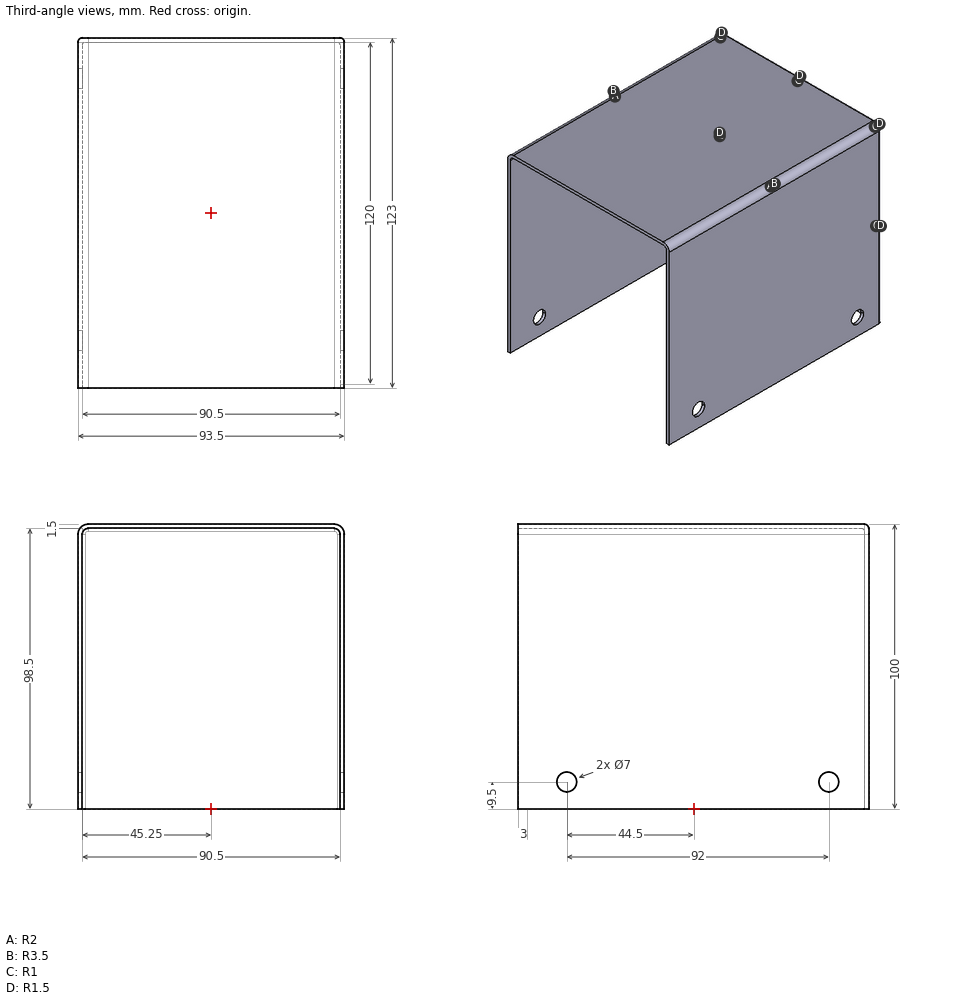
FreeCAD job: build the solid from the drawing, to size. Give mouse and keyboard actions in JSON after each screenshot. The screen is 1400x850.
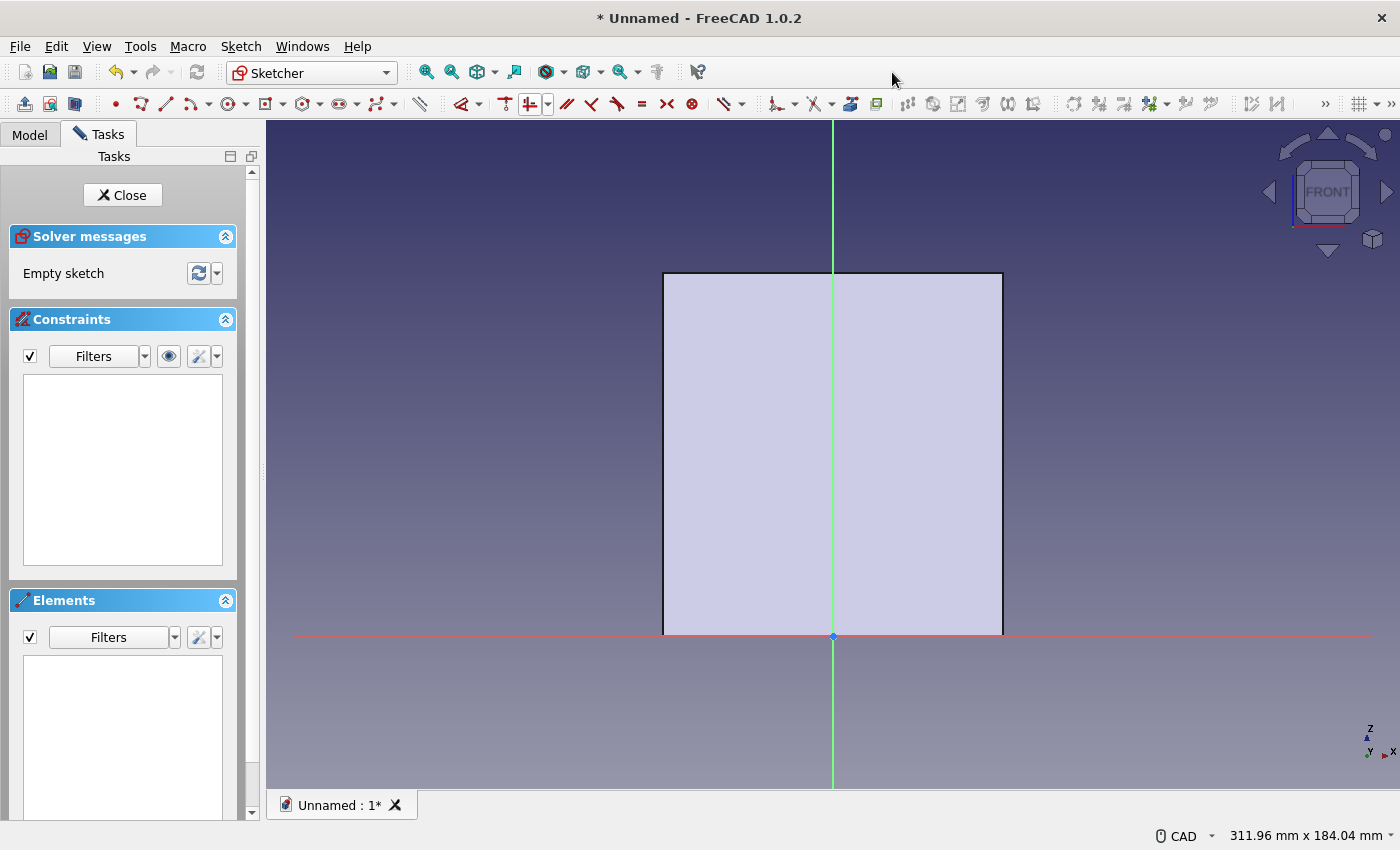
{"action": "key", "text": "g r"}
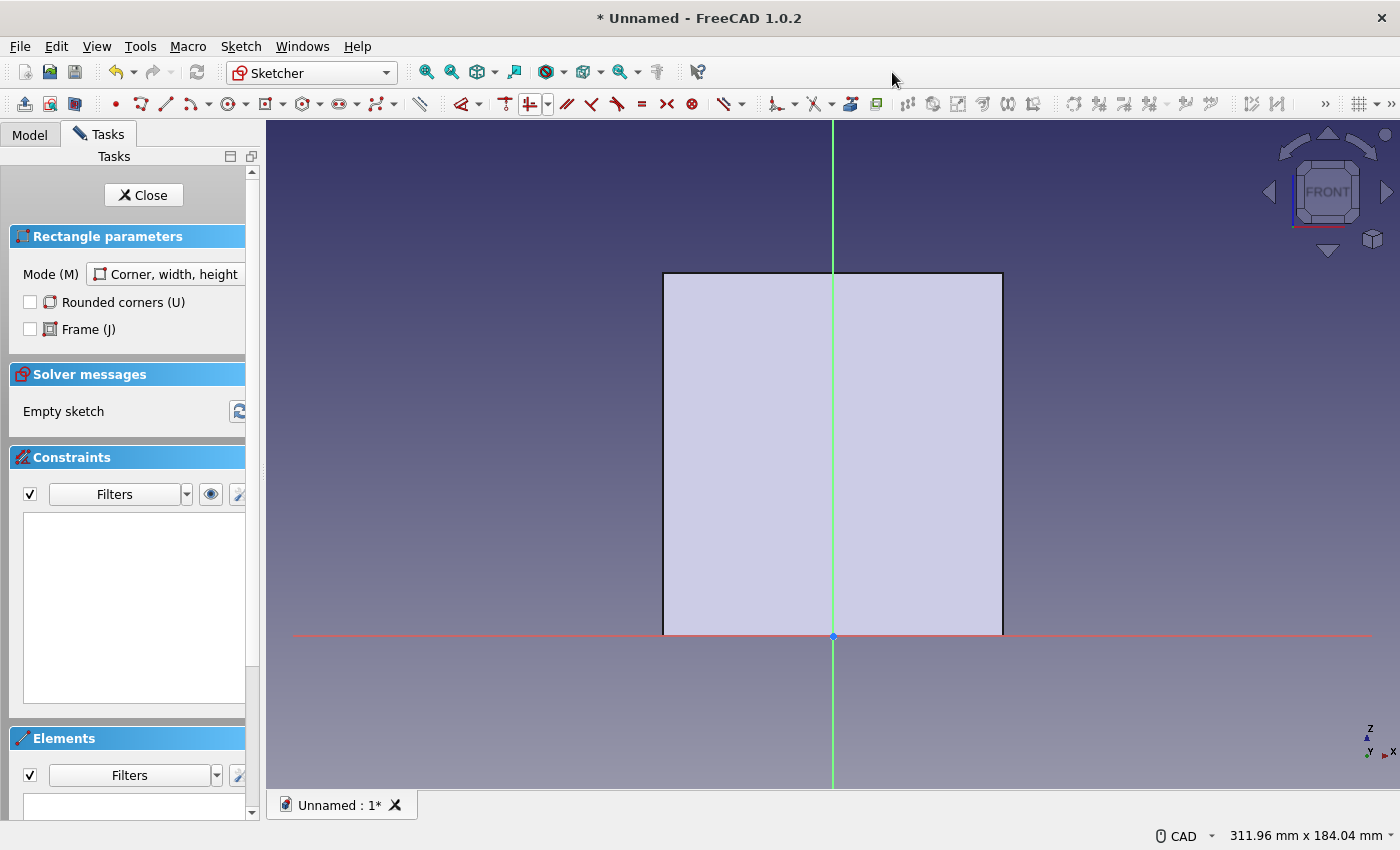
{"action": "left_click", "coordinate": [669, 278]}
{"action": "left_click", "coordinate": [997, 636]}
{"action": "key", "text": "Escape"}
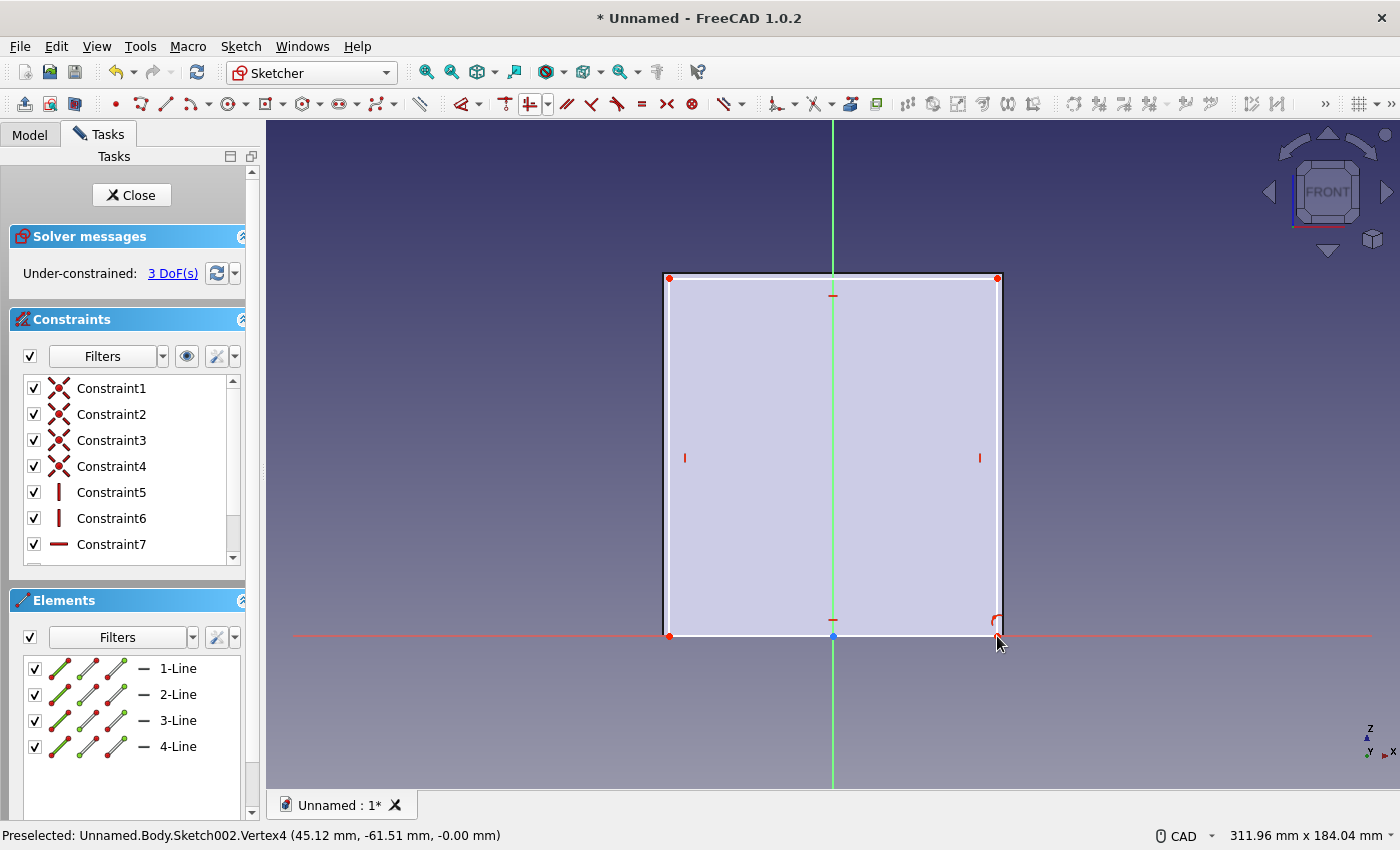
{"action": "left_click", "coordinate": [460, 104]}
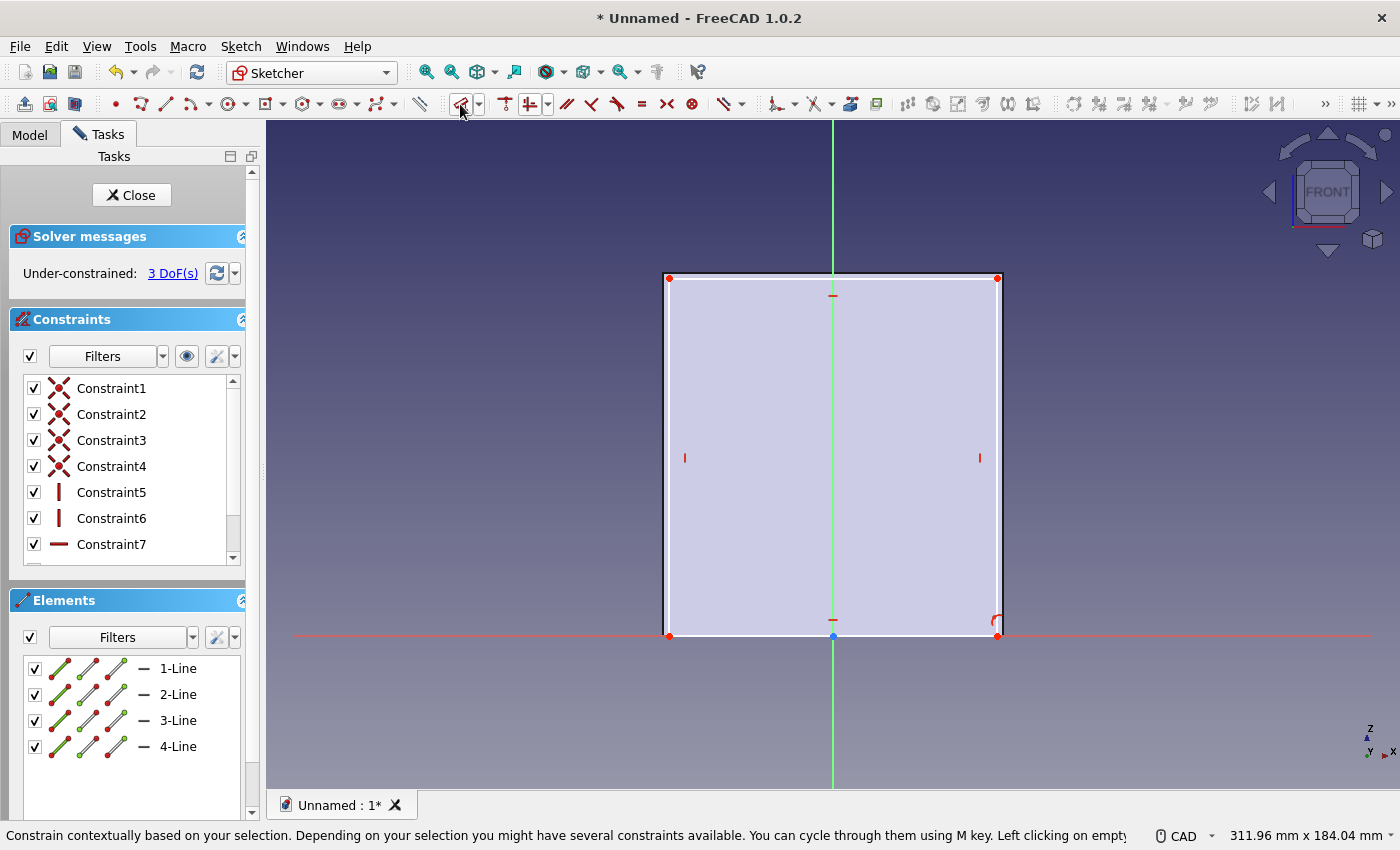
{"action": "left_click", "coordinate": [669, 386]}
{"action": "left_click", "coordinate": [635, 458]}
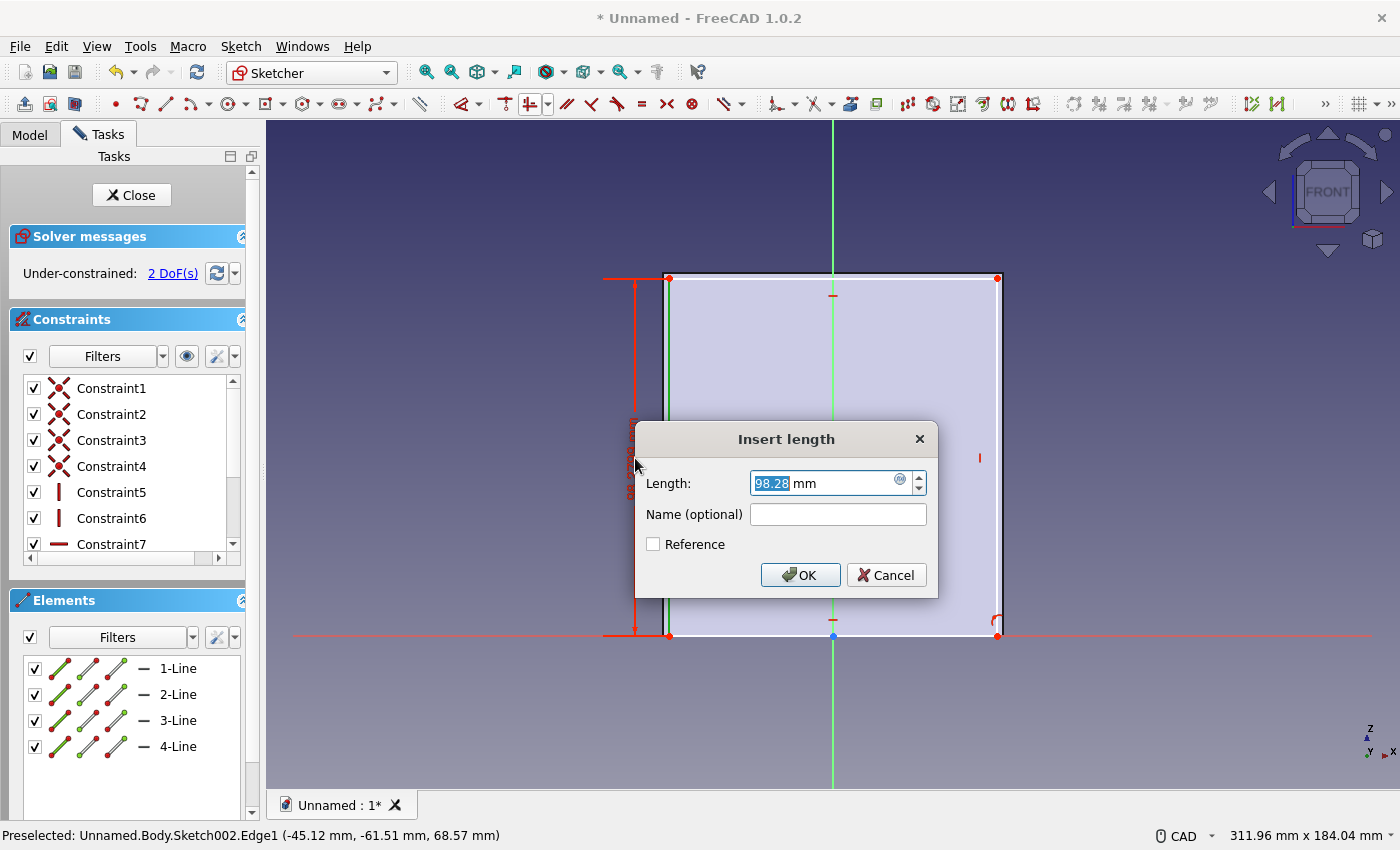
{"action": "type", "text": "98.5"}
{"action": "key", "text": "Return"}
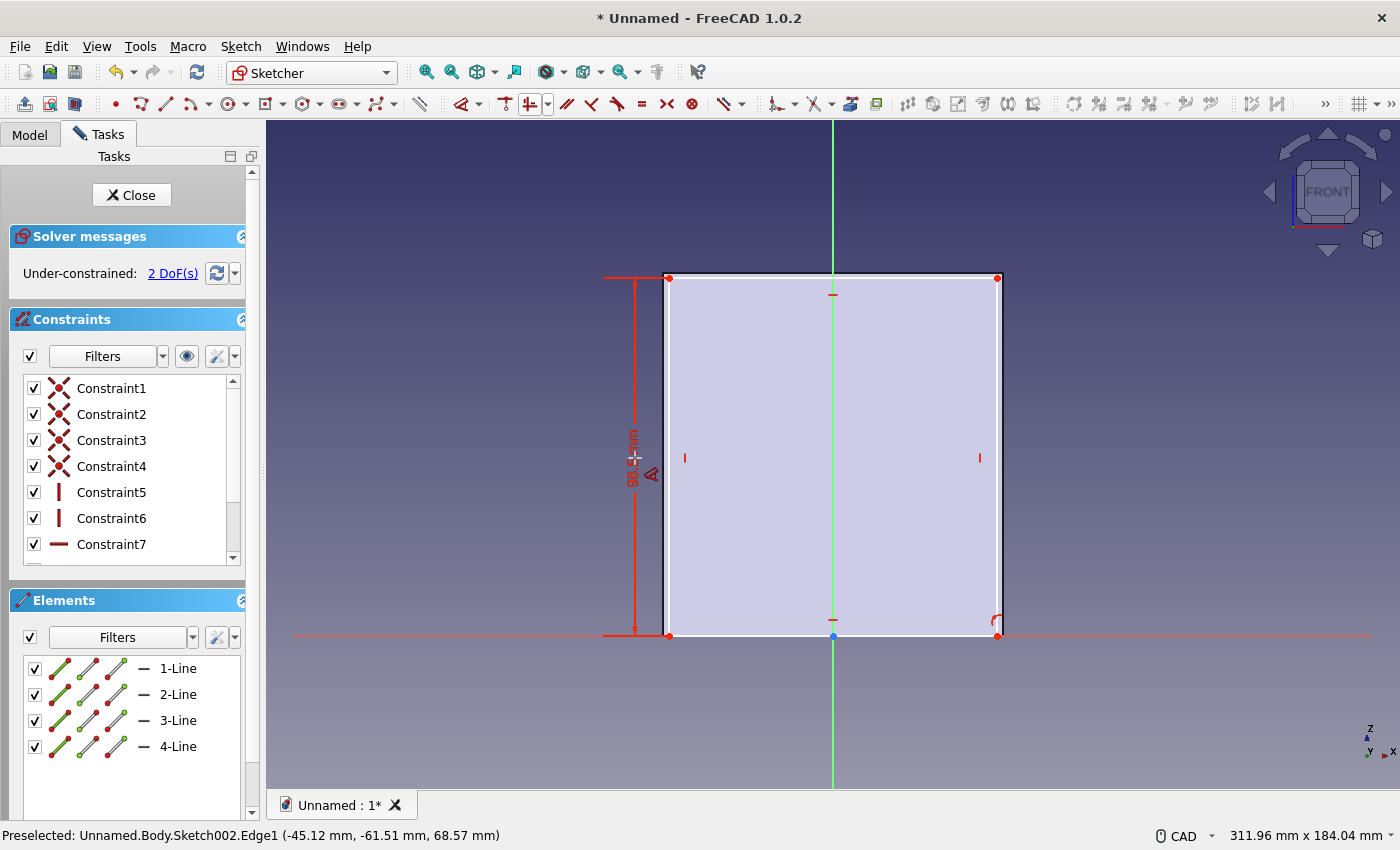
{"action": "left_click", "coordinate": [767, 636]}
{"action": "left_click", "coordinate": [758, 670]}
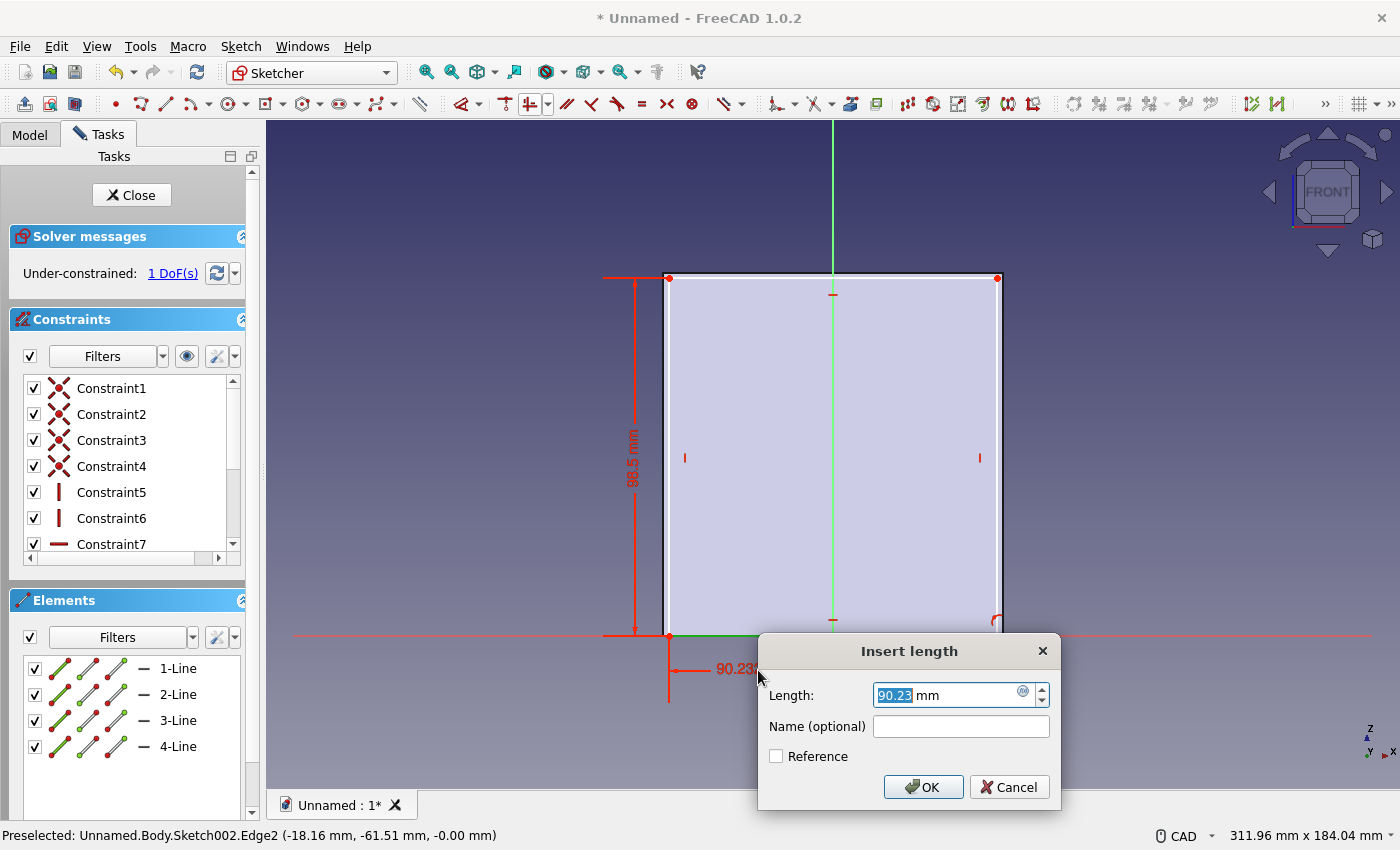
{"action": "type", "text": "90.5"}
{"action": "key", "text": "Return"}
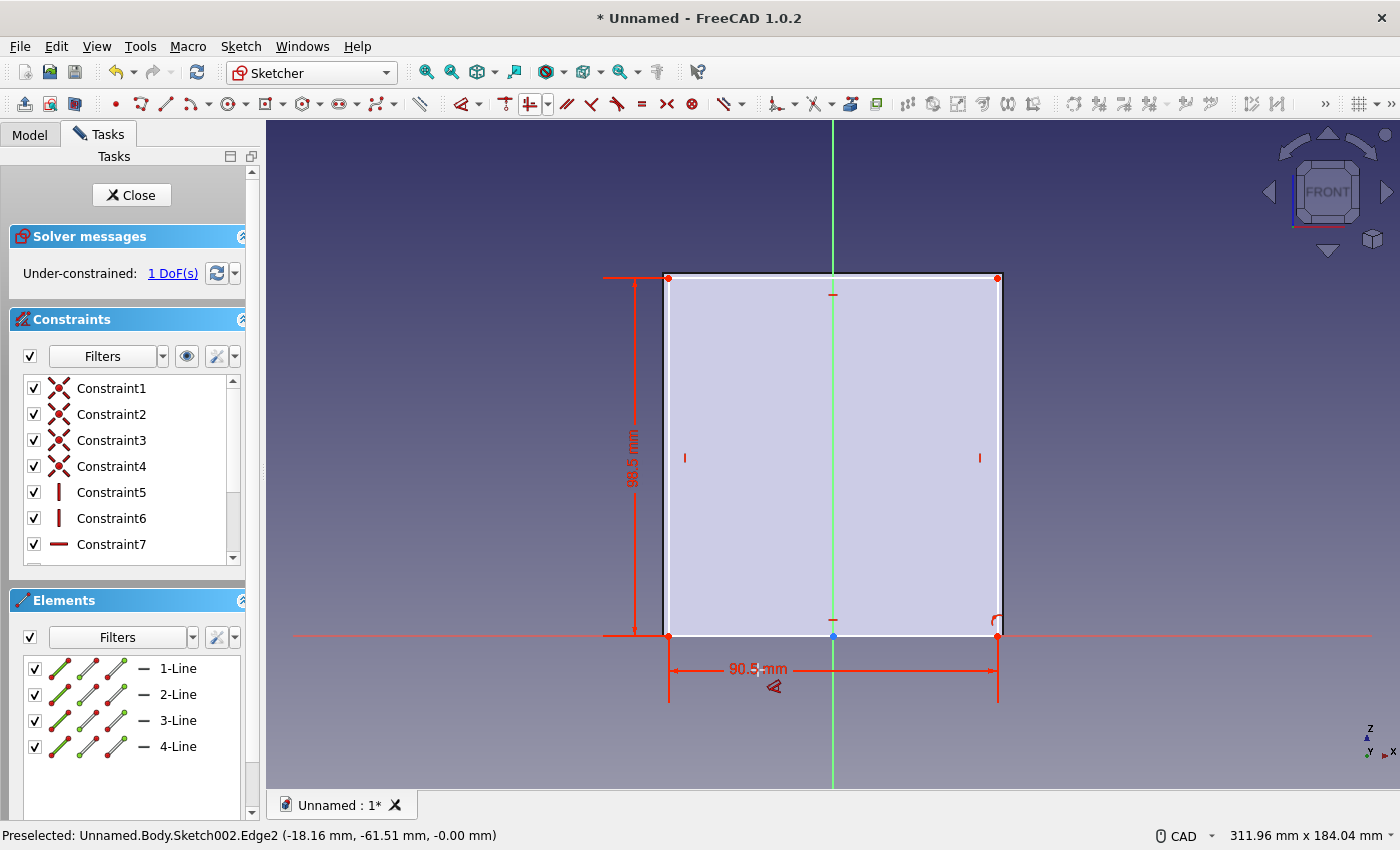
{"action": "left_click", "coordinate": [669, 278]}
{"action": "left_click", "coordinate": [751, 244]}